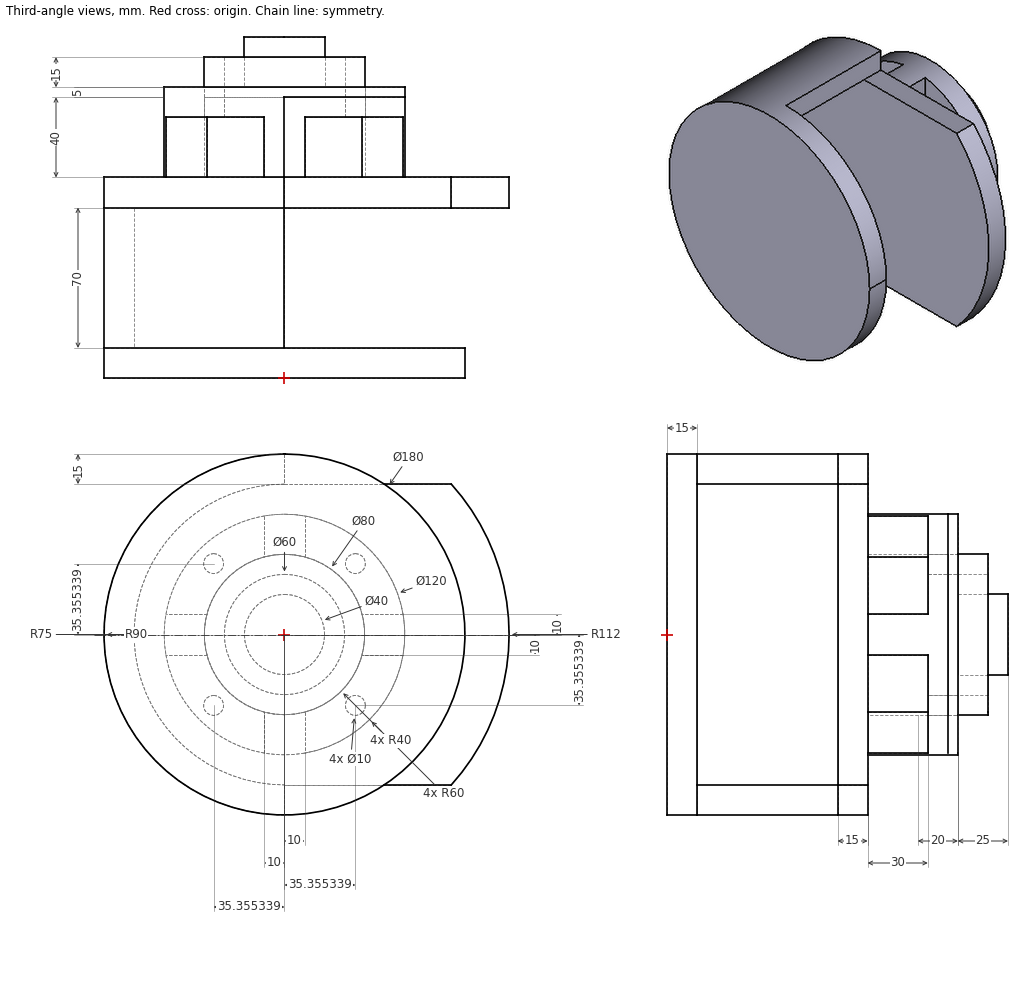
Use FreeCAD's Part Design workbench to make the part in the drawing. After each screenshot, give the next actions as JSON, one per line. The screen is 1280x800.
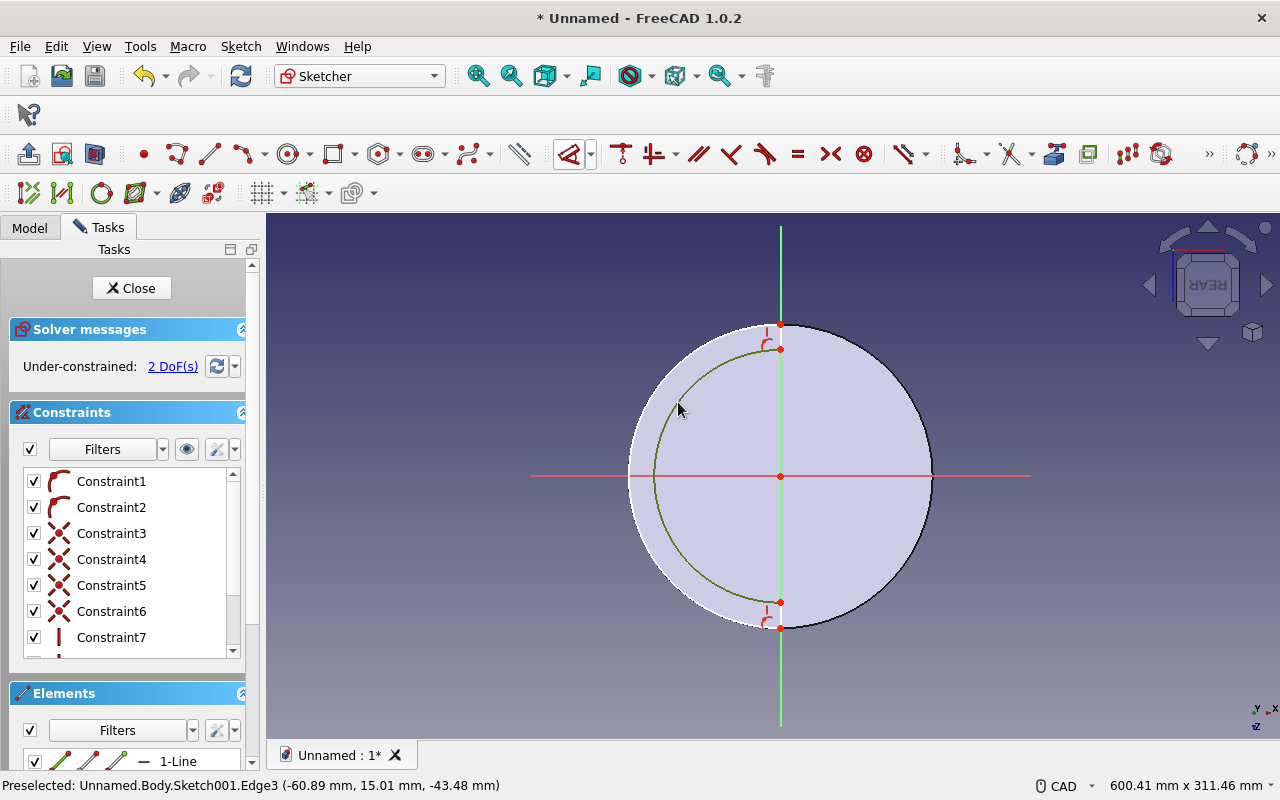
{"action": "key", "text": "k r"}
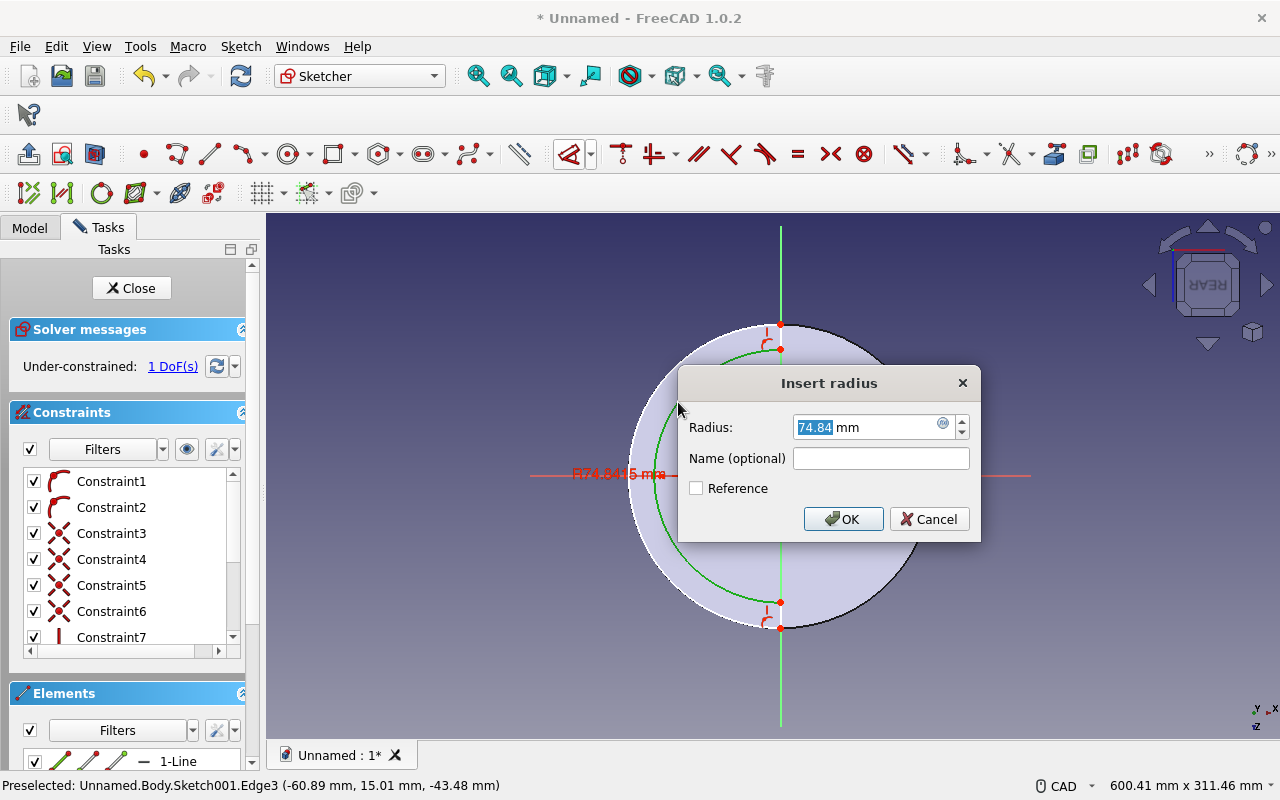
{"action": "type", "text": "75"}
{"action": "key", "text": "Return"}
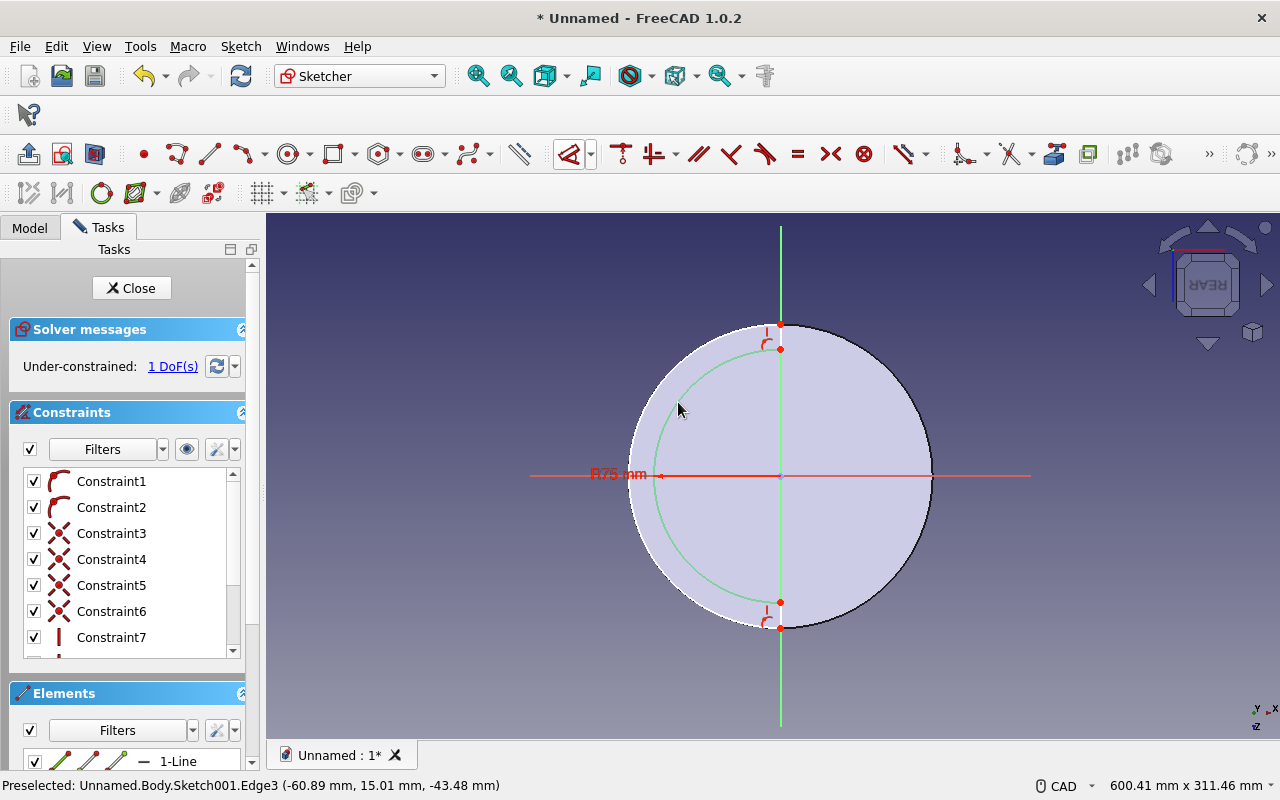
{"action": "left_click", "coordinate": [658, 387]}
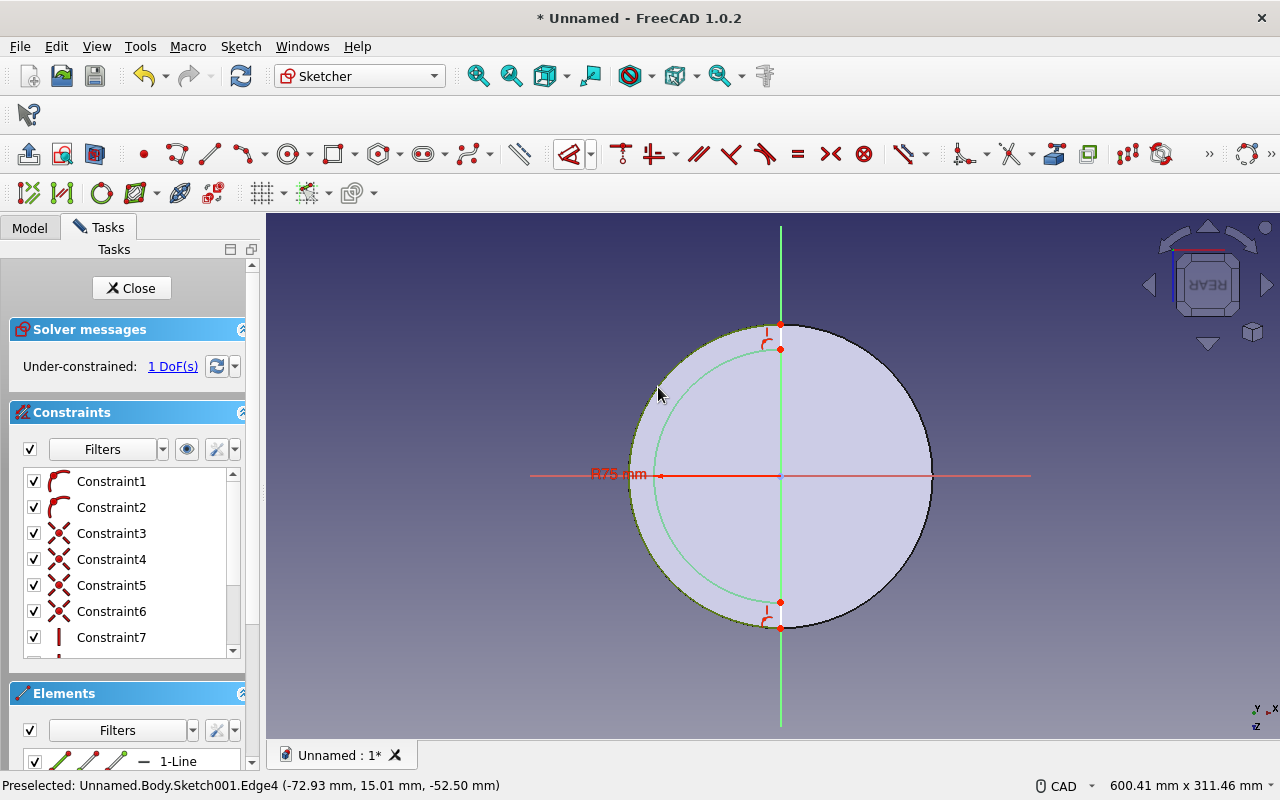
{"action": "key", "text": "k r"}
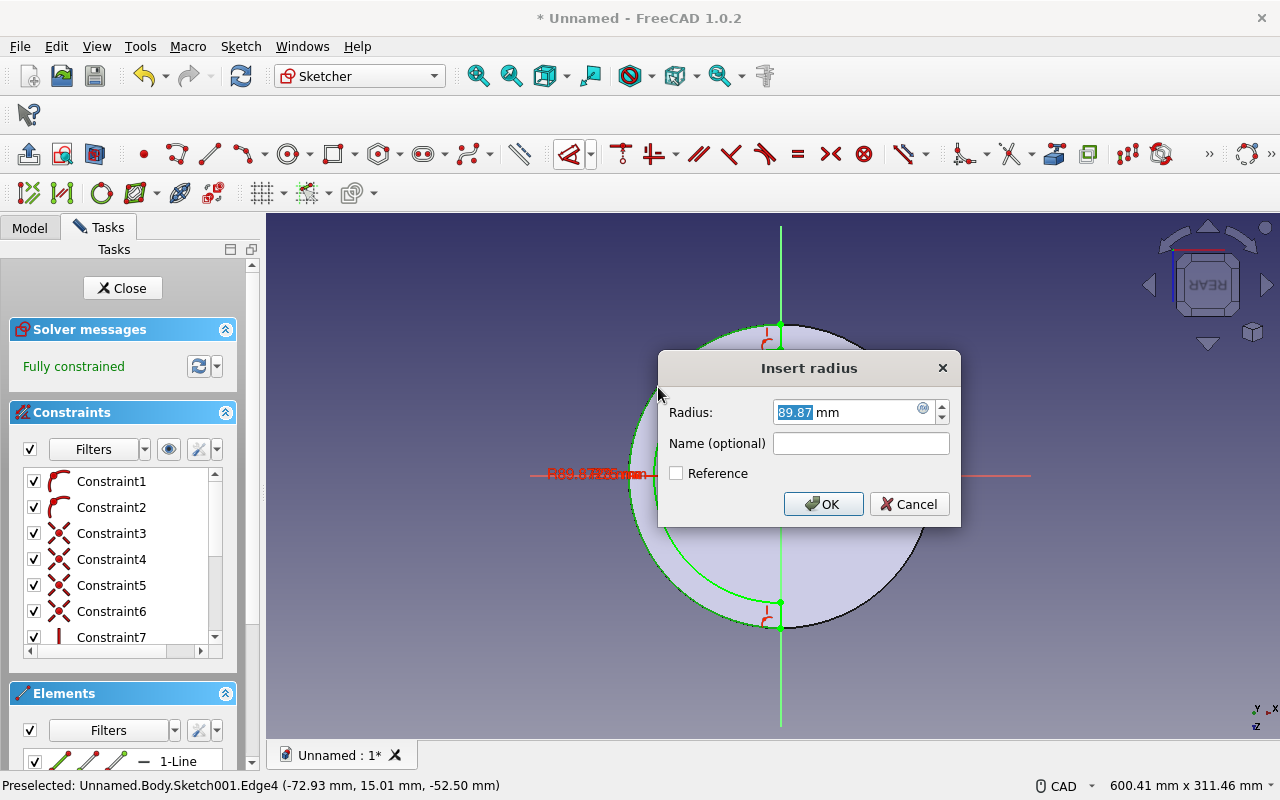
{"action": "type", "text": "90"}
{"action": "key", "text": "Return"}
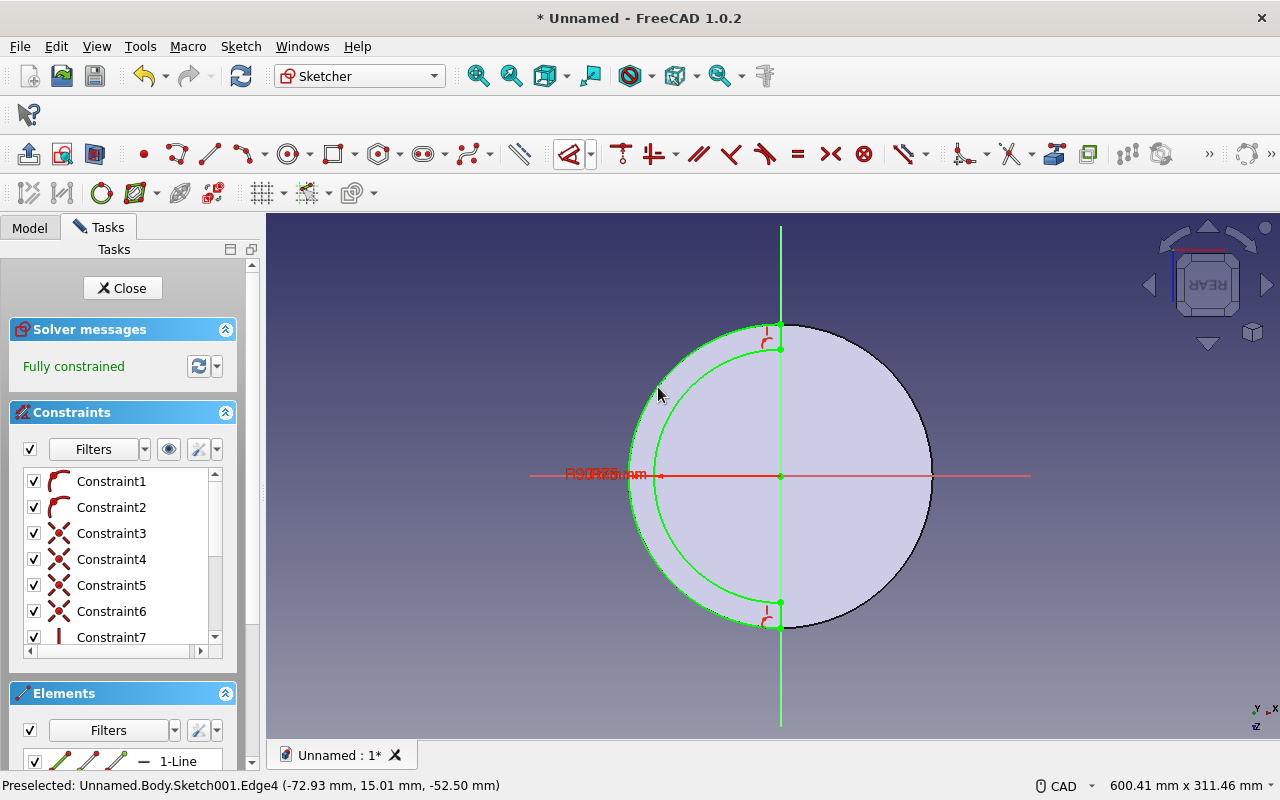
{"action": "left_click", "coordinate": [123, 288]}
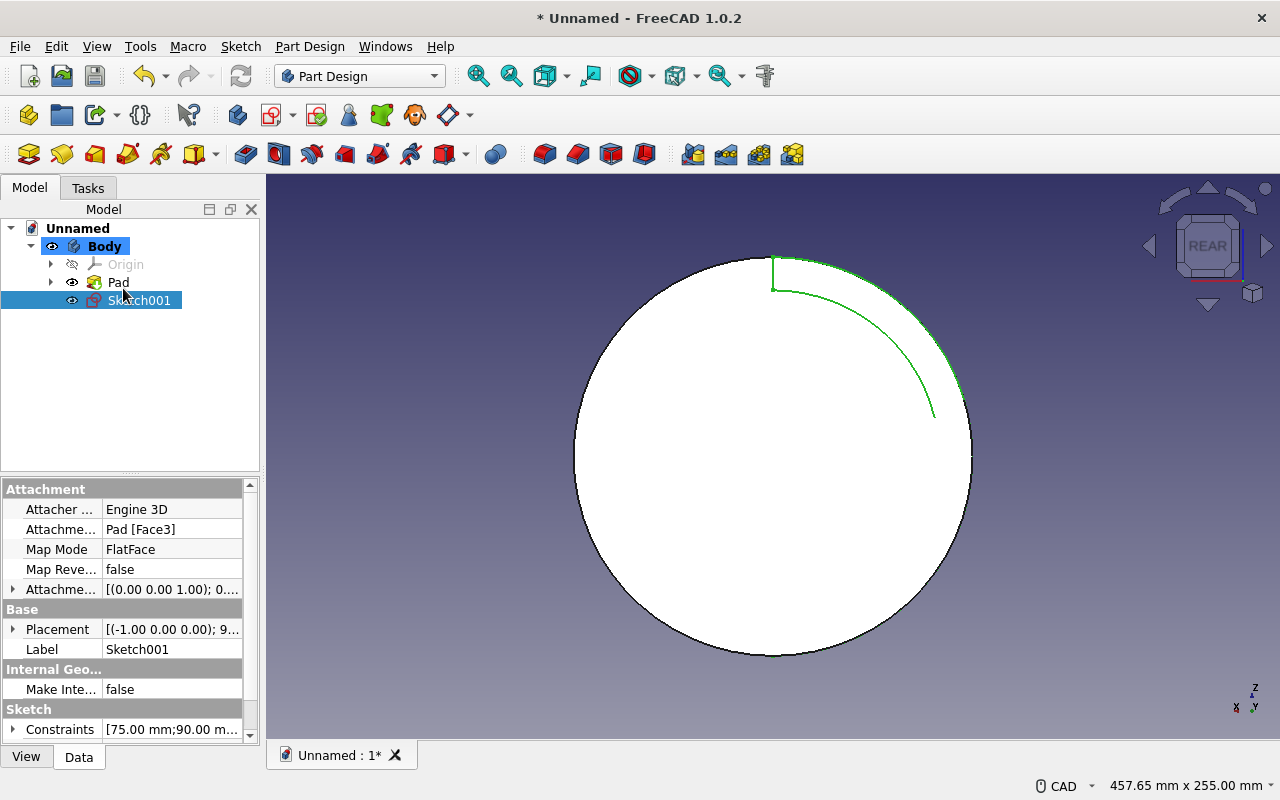
{"action": "left_click", "coordinate": [29, 154]}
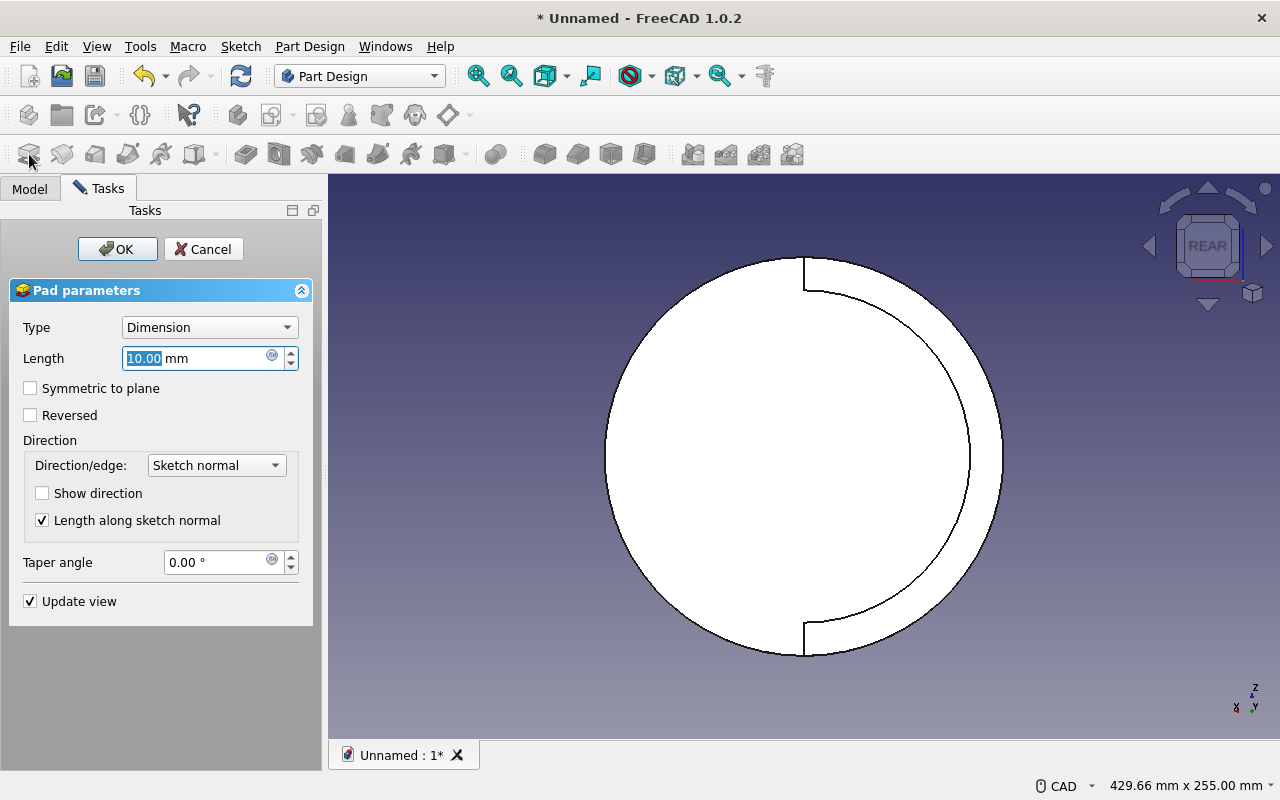
{"action": "type", "text": "70"}
{"action": "key", "text": "Tab"}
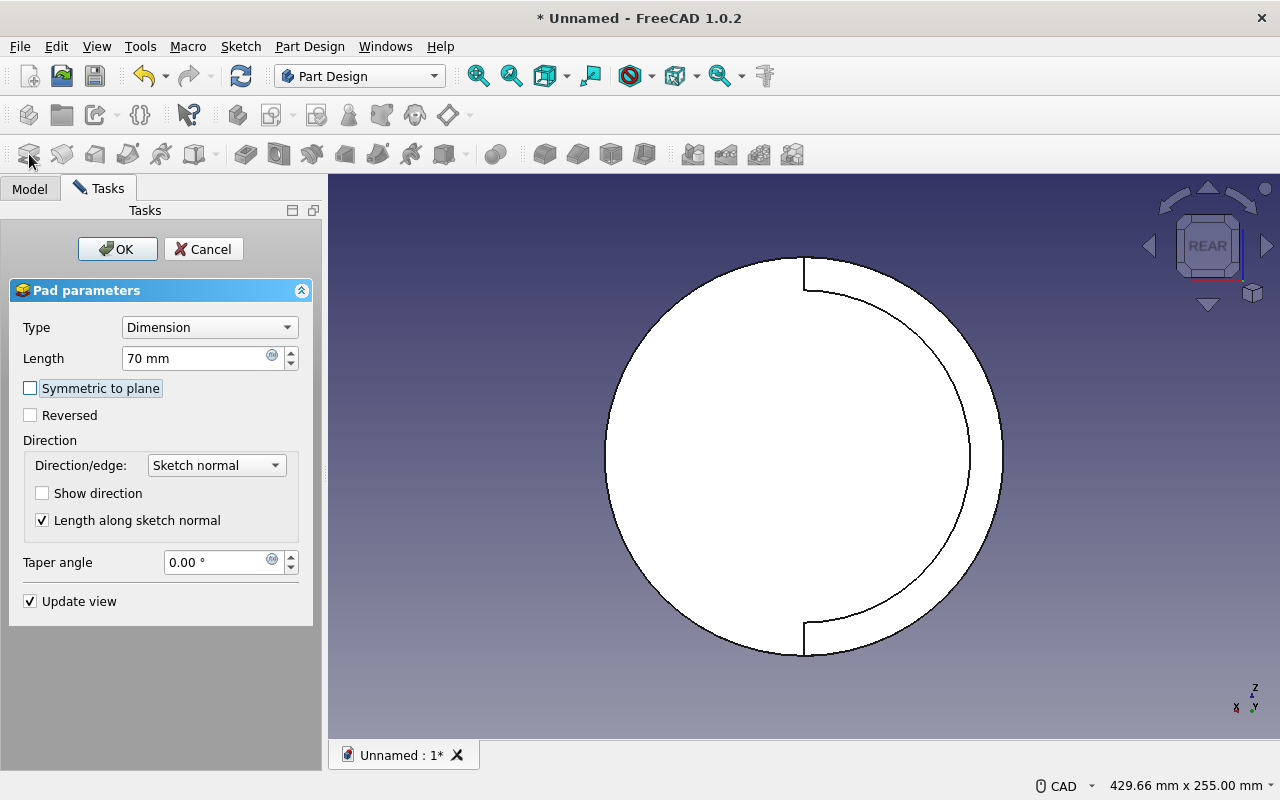
{"action": "left_click", "coordinate": [118, 249]}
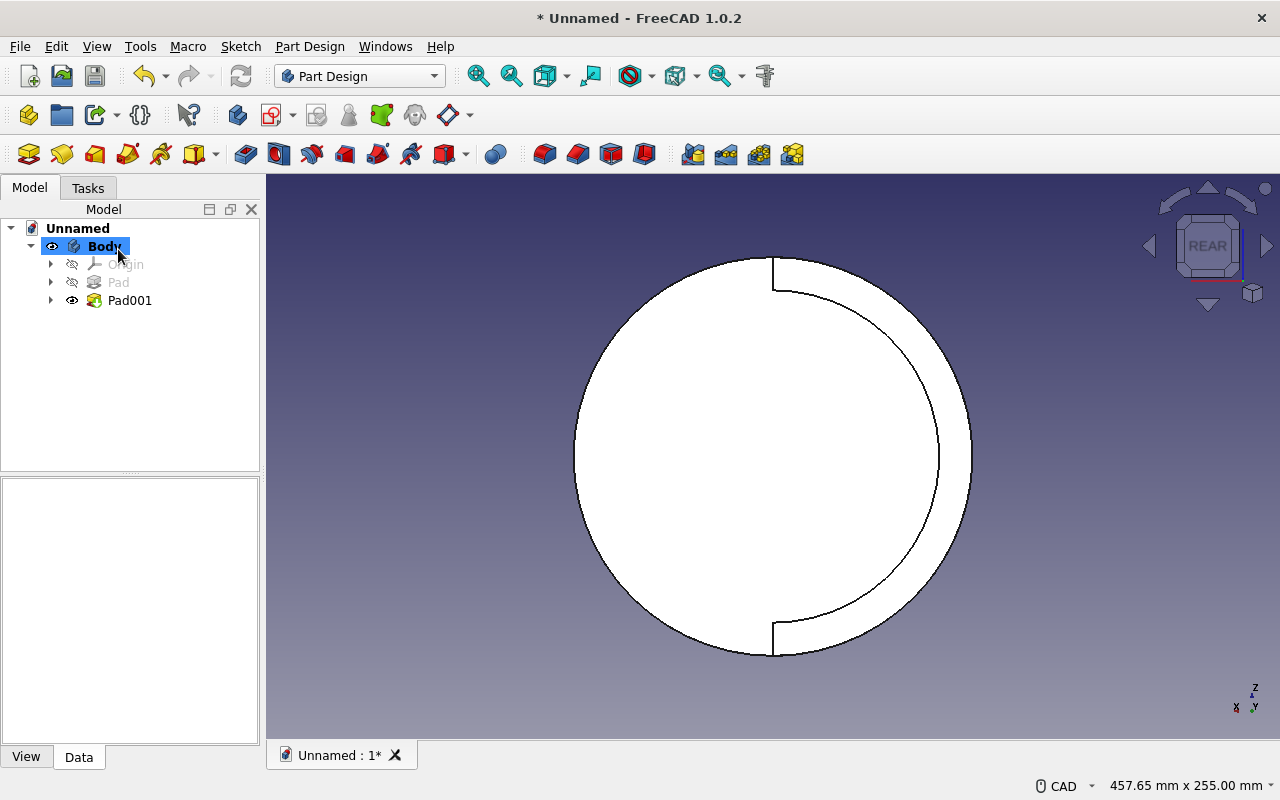
{"action": "left_click", "coordinate": [844, 285]}